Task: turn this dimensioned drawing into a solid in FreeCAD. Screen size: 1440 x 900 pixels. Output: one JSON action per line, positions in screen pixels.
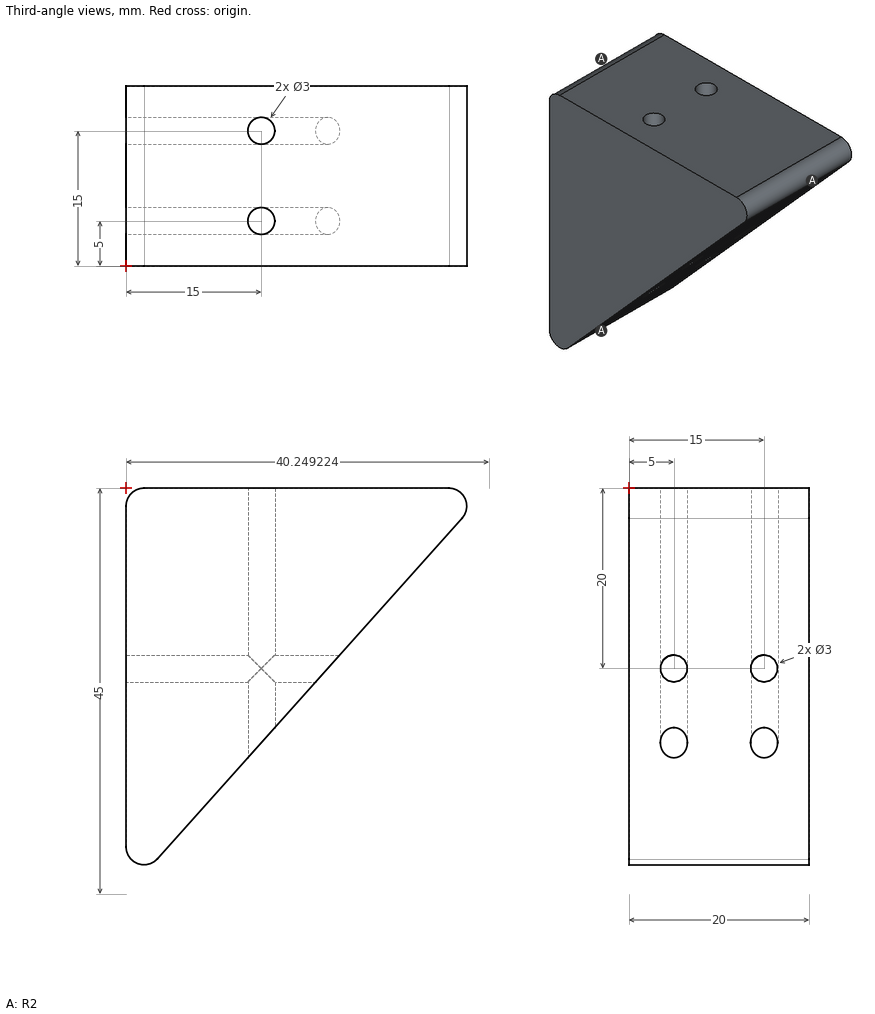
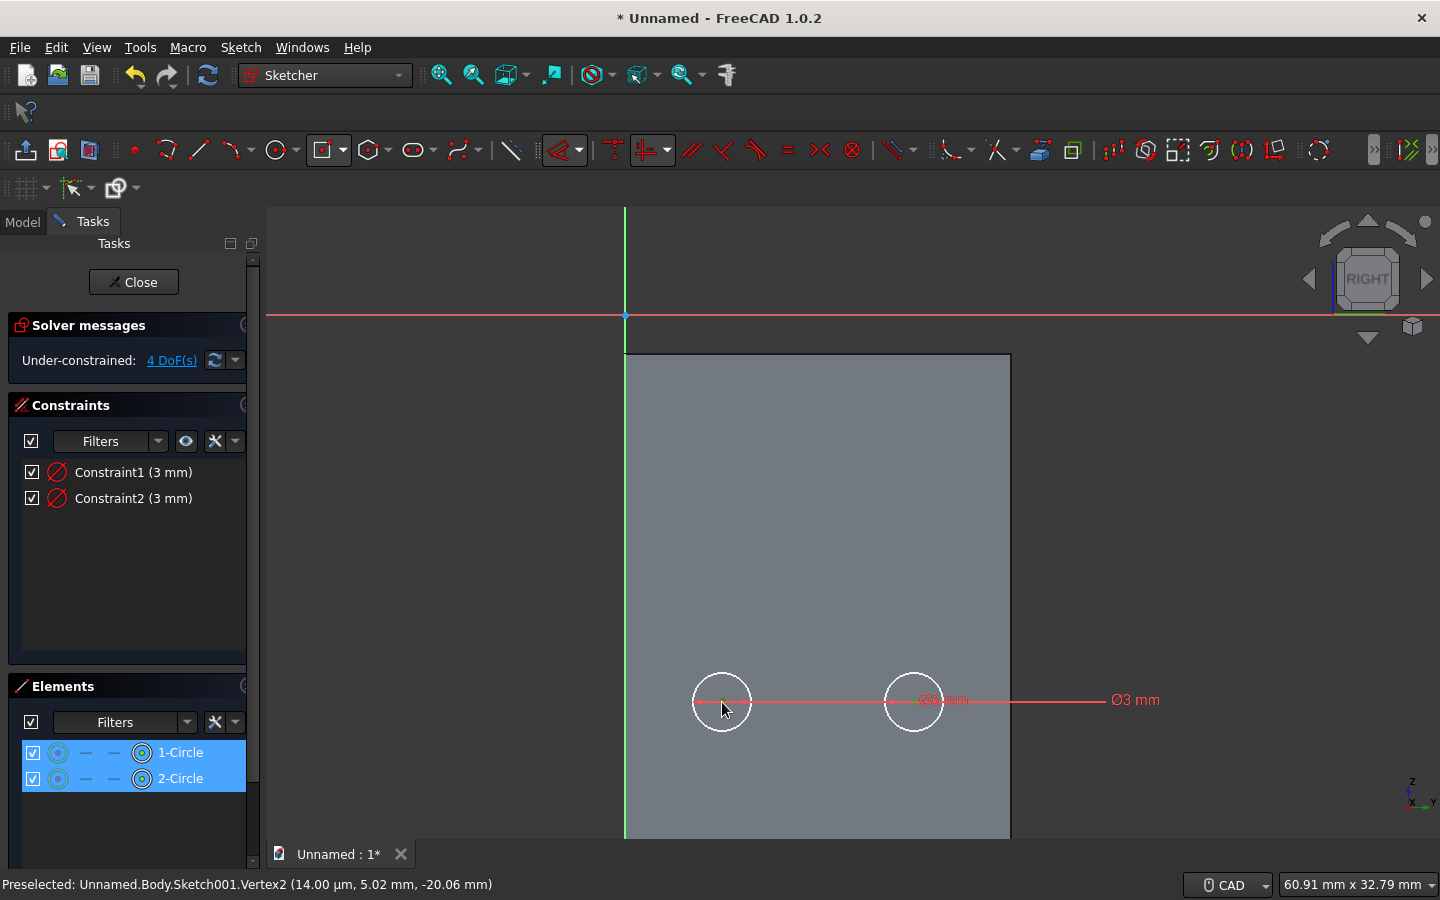
{"action": "key", "text": "h"}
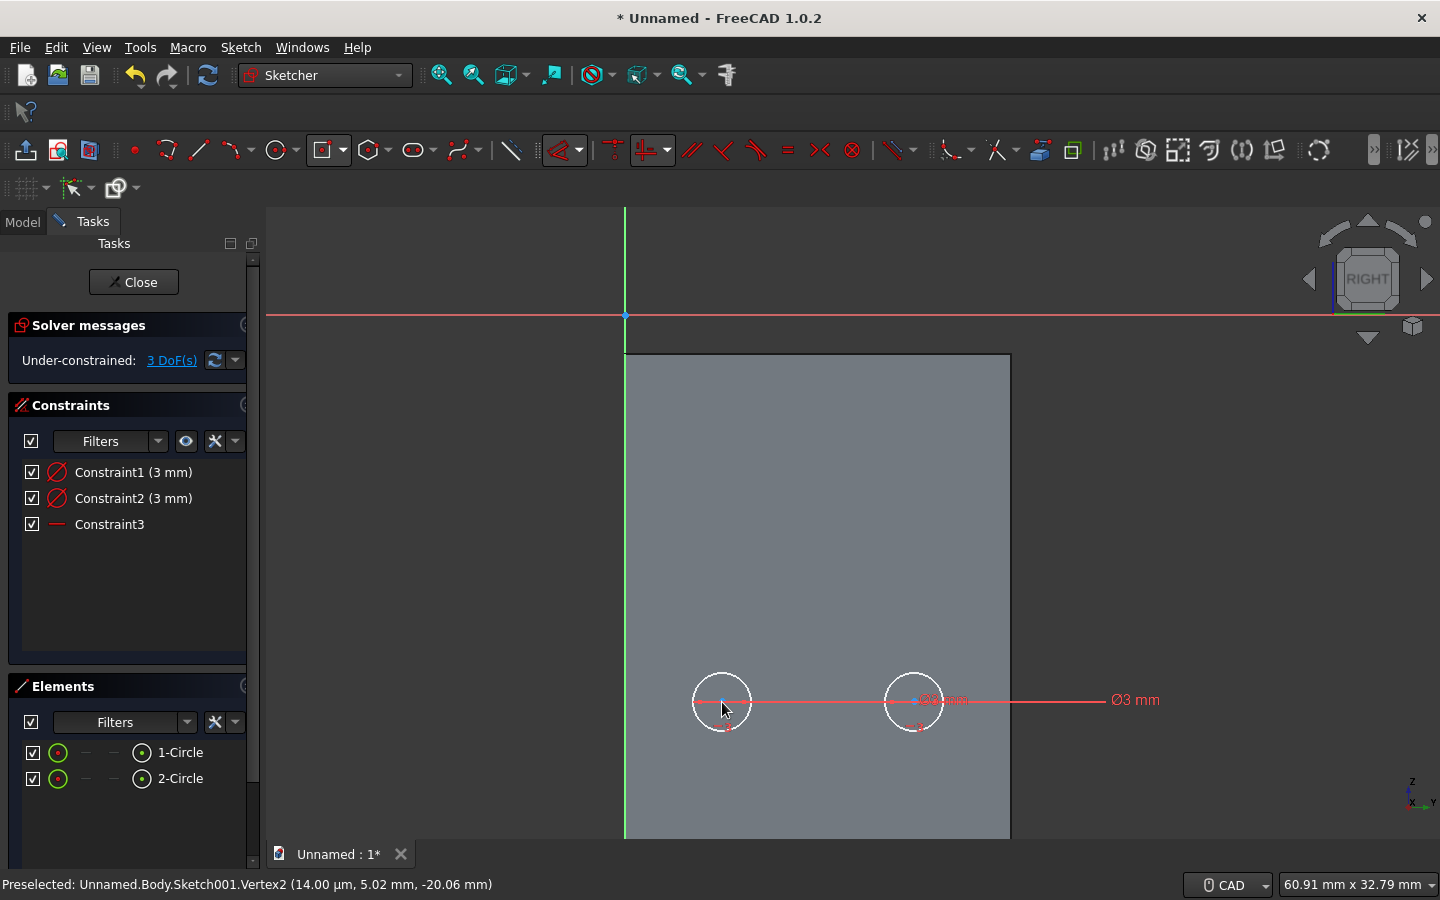
{"action": "key", "text": "d"}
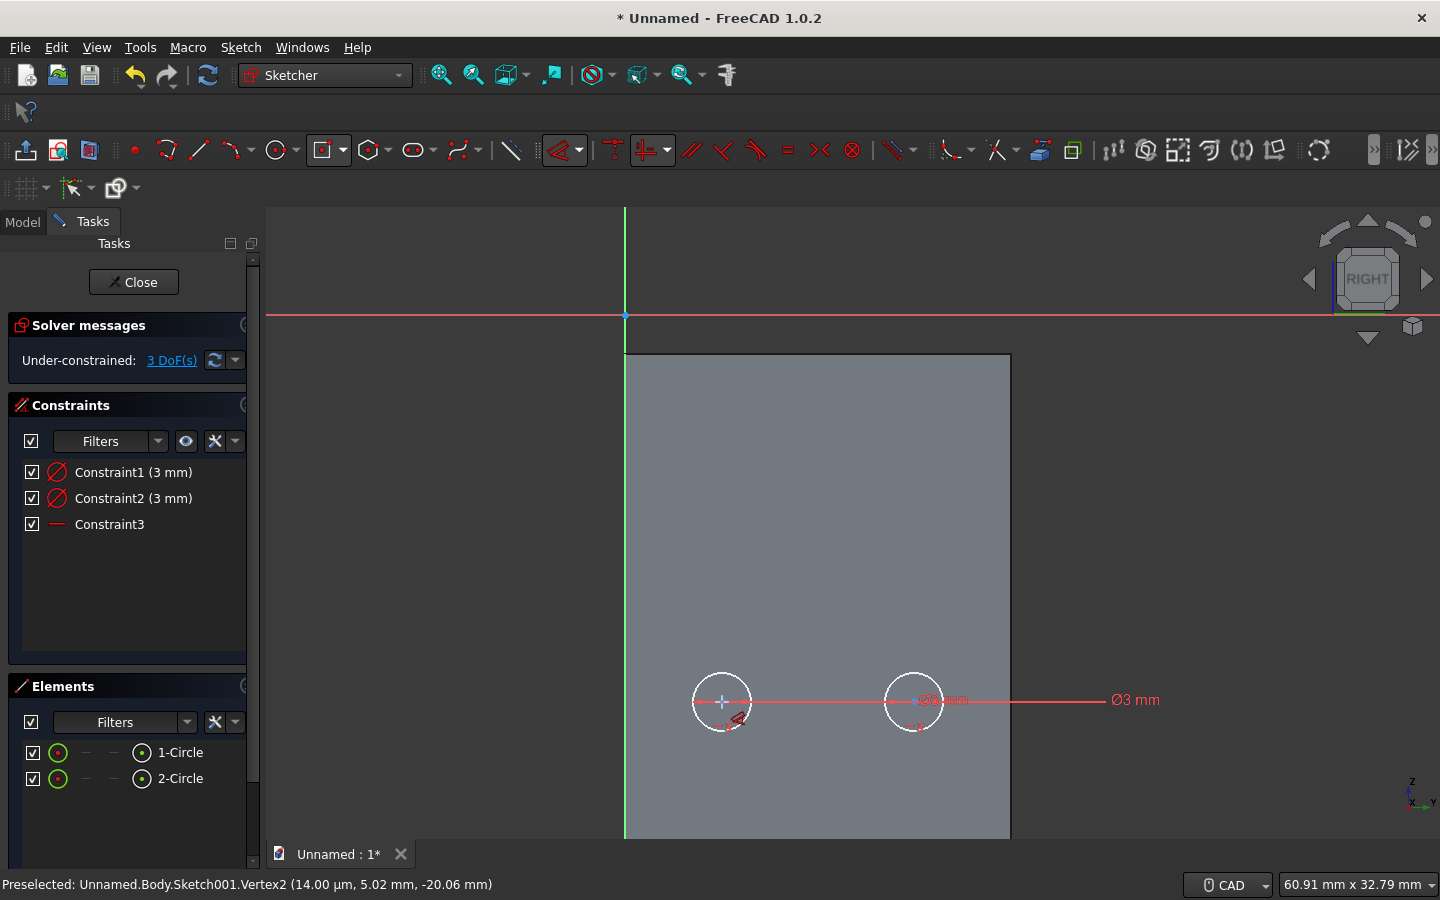
{"action": "left_click", "coordinate": [722, 702]}
{"action": "left_click", "coordinate": [674, 281]}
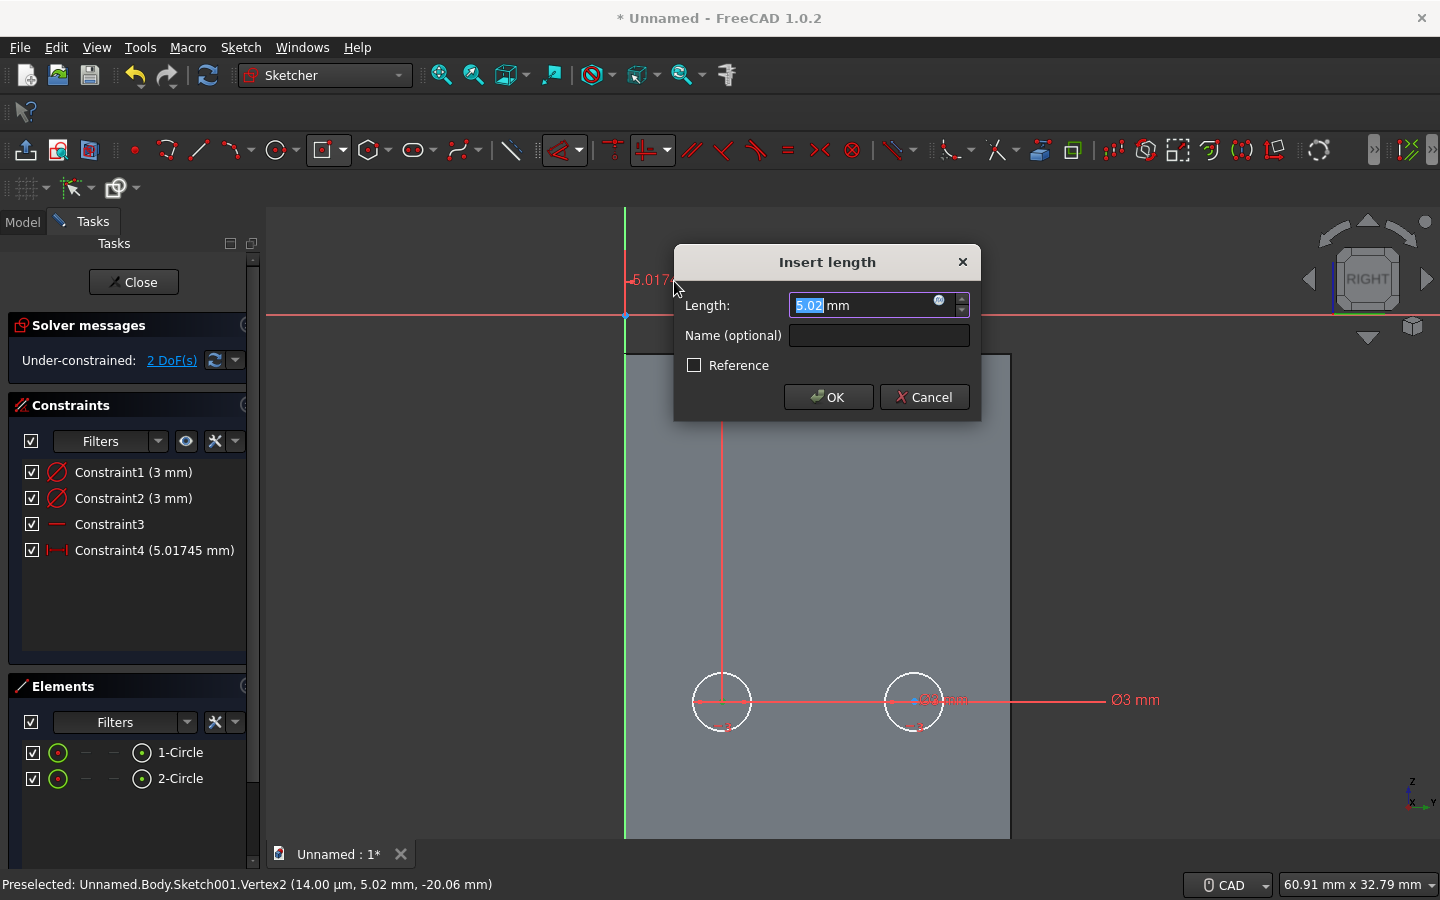
{"action": "type", "text": "5"}
{"action": "key", "text": "Return"}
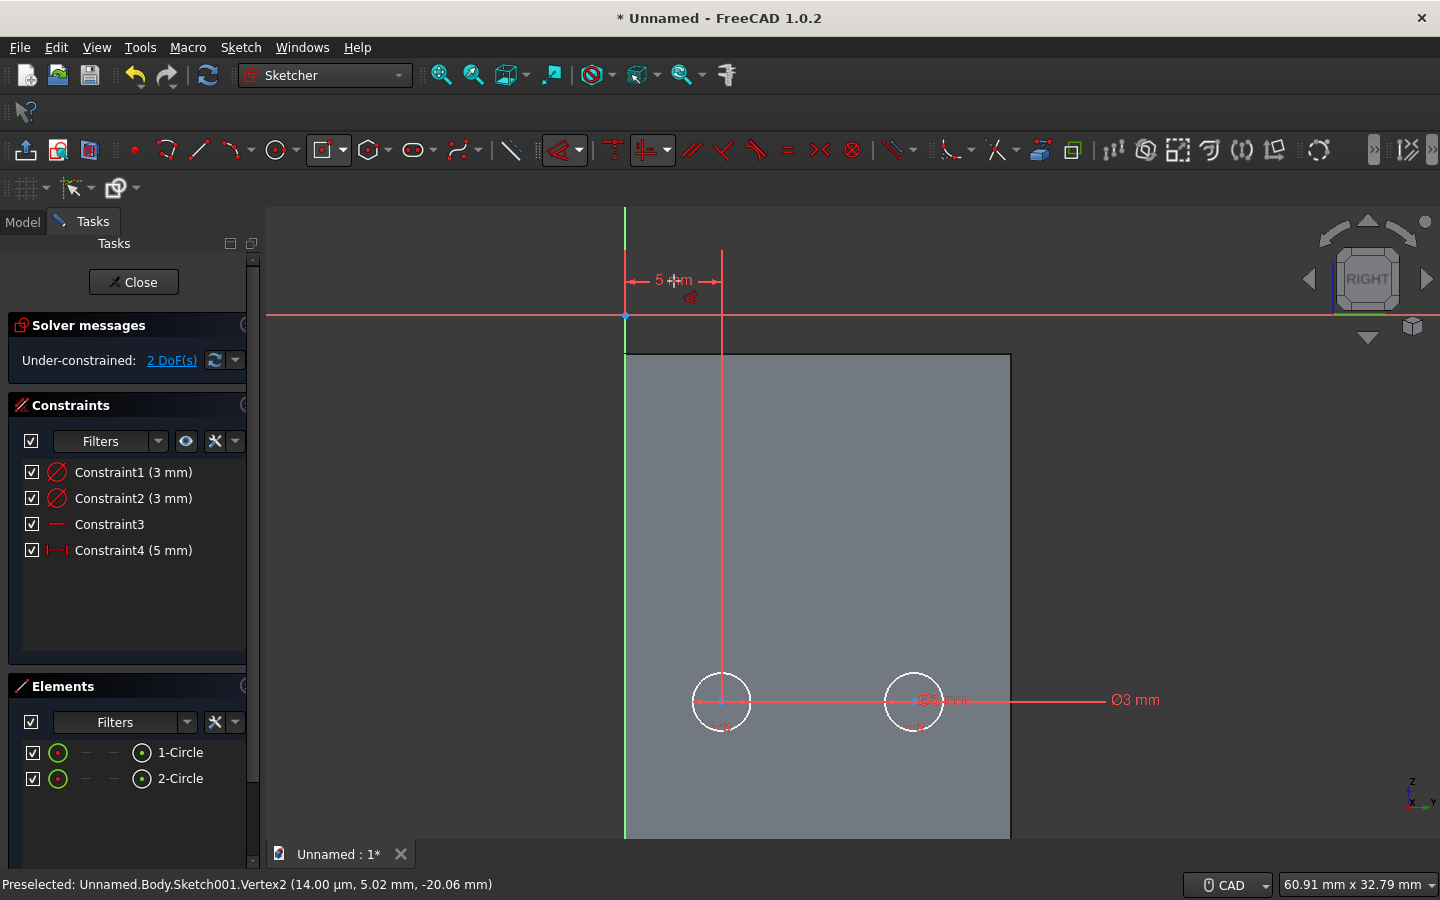
{"action": "left_click", "coordinate": [914, 702]}
{"action": "left_click", "coordinate": [770, 281]}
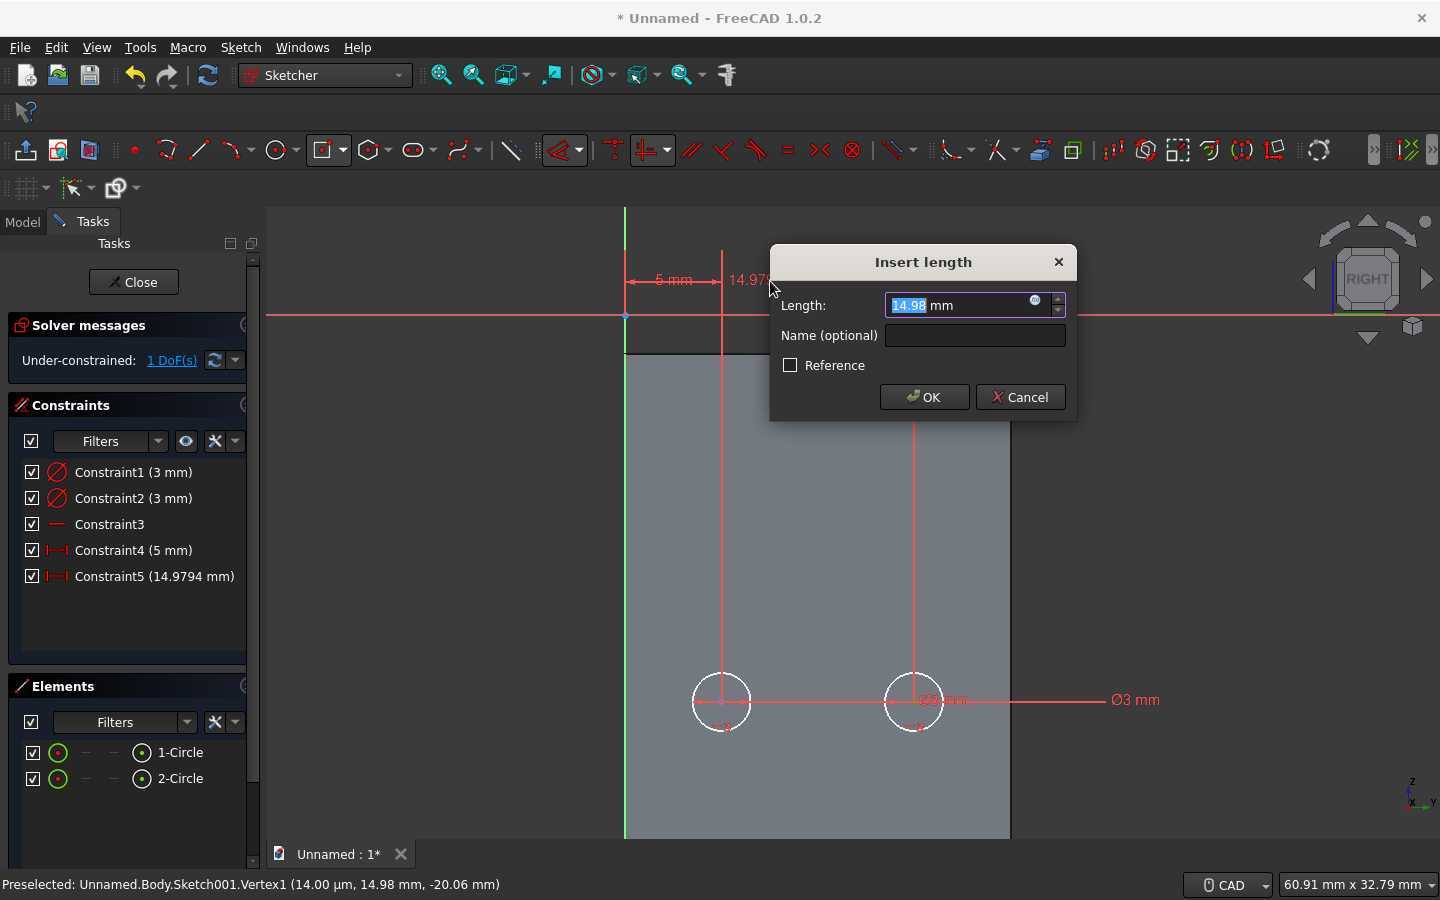
{"action": "type", "text": "15"}
{"action": "key", "text": "Return"}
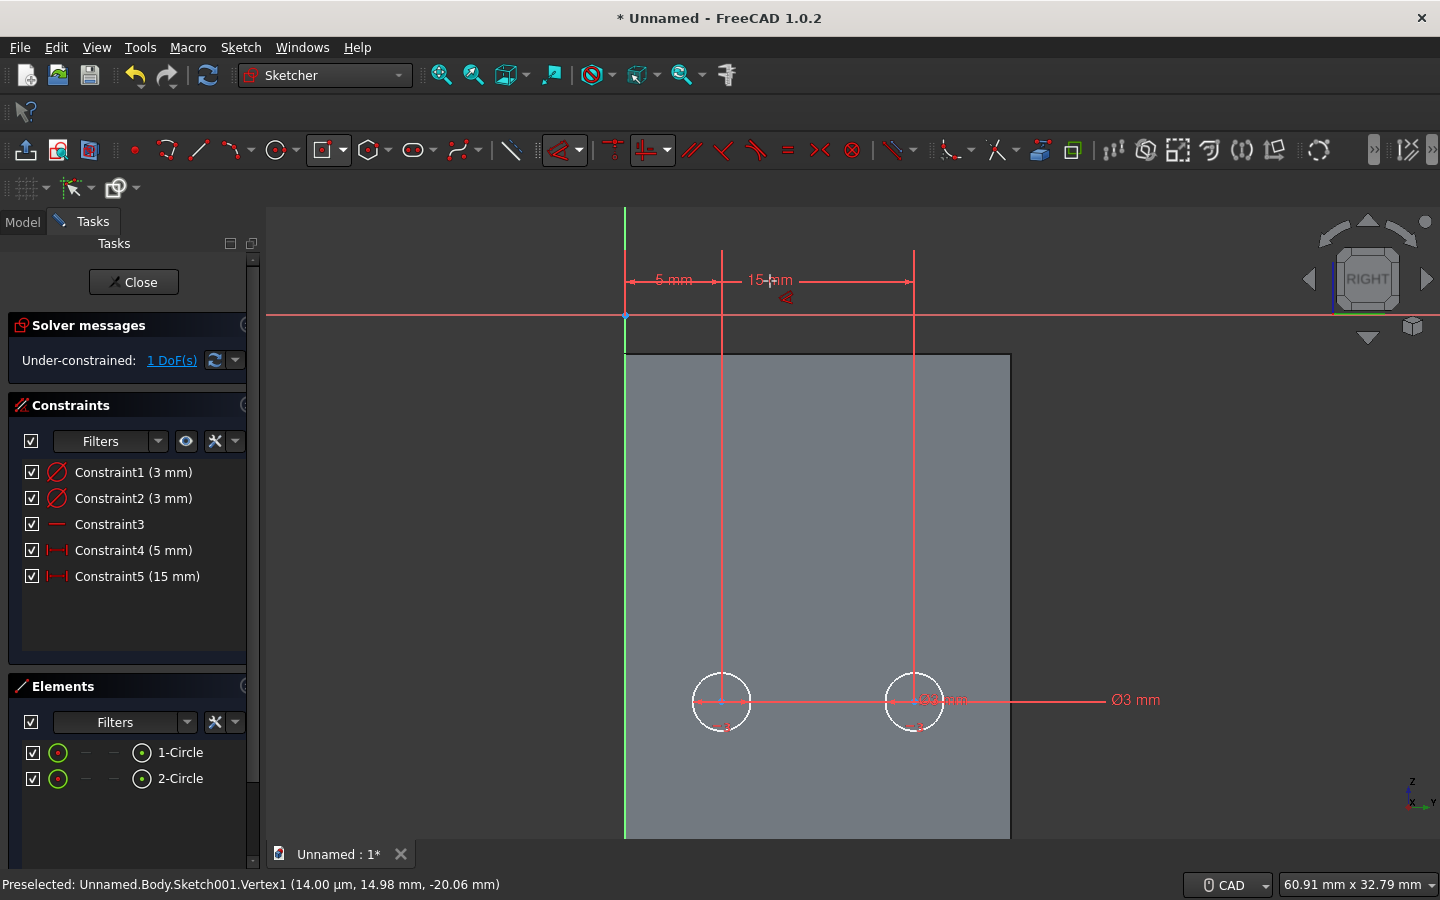
{"action": "left_click", "coordinate": [914, 702]}
{"action": "left_click", "coordinate": [591, 509]}